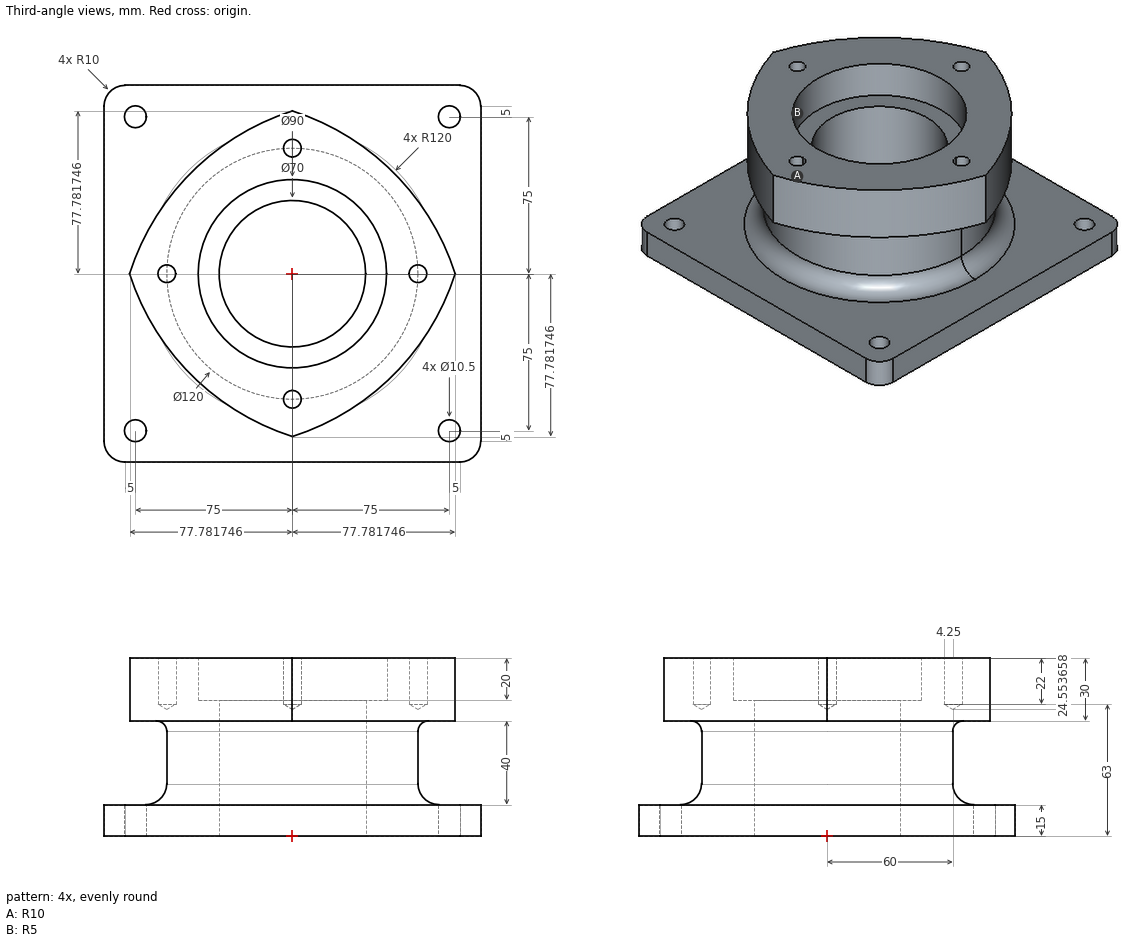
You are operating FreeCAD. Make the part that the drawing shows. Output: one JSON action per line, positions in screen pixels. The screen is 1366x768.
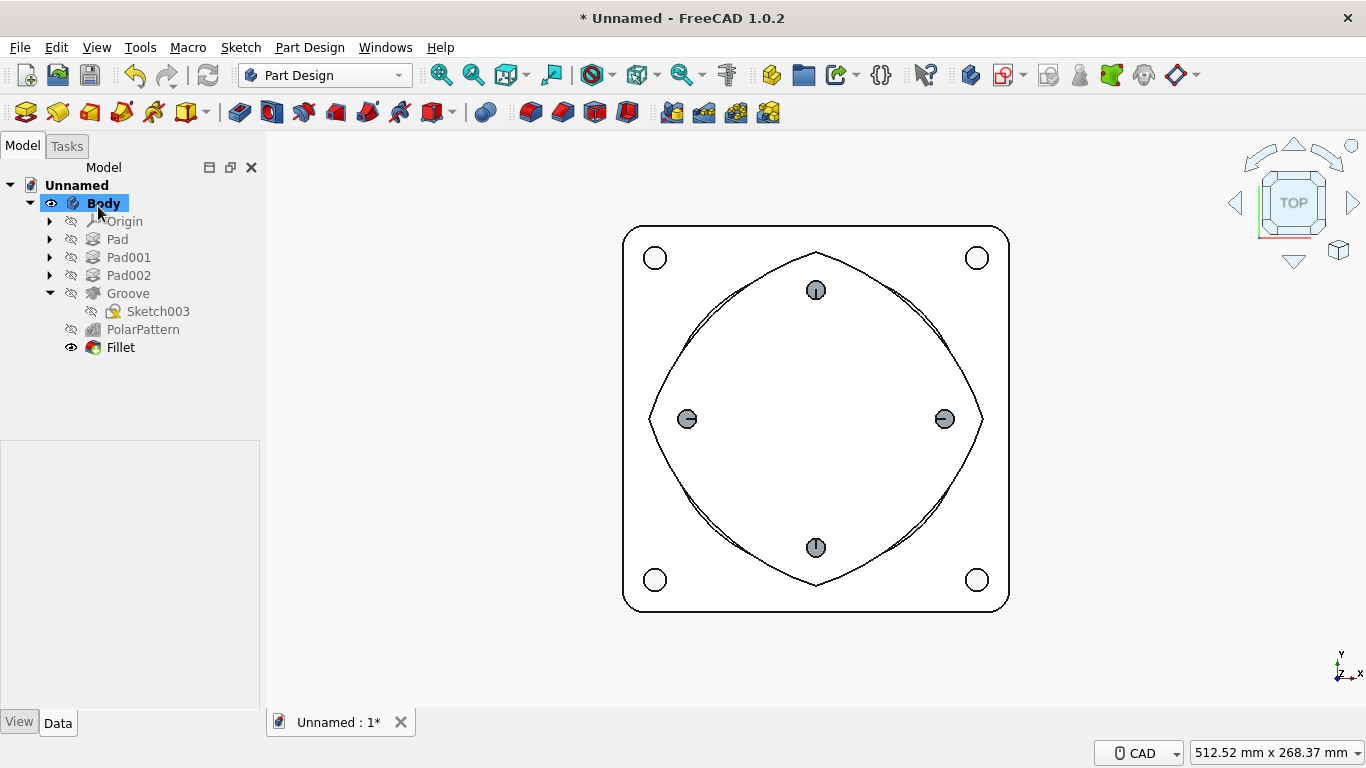
{"action": "key", "text": "0"}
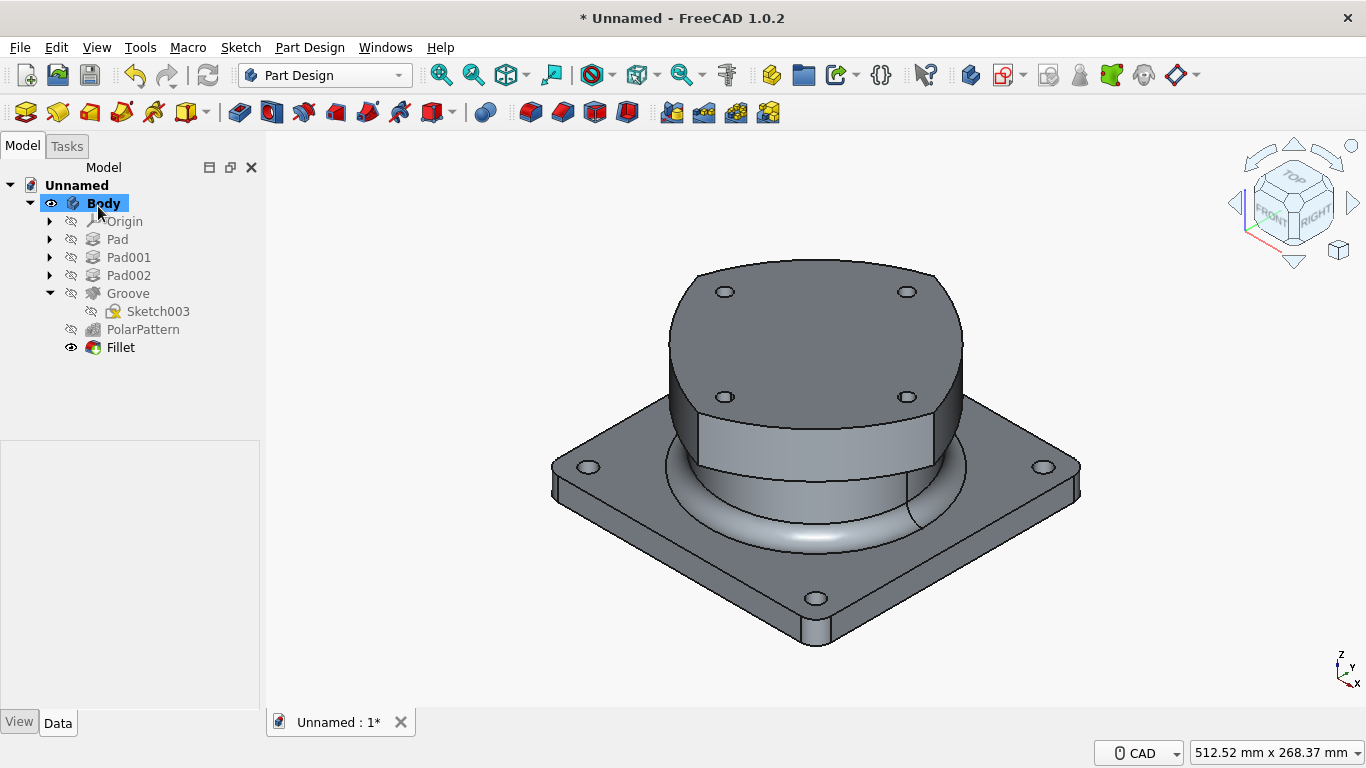
{"action": "key", "text": "1"}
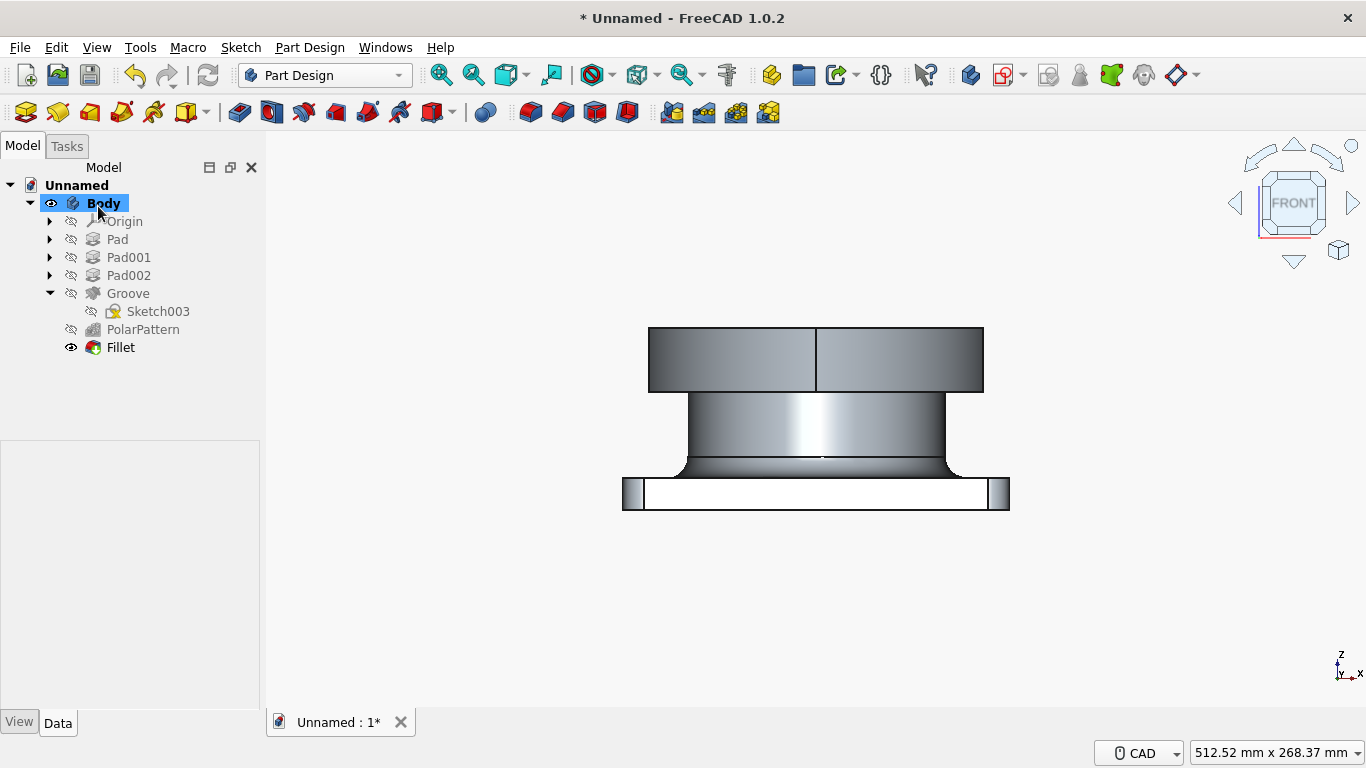
{"action": "left_click", "coordinate": [442, 76]}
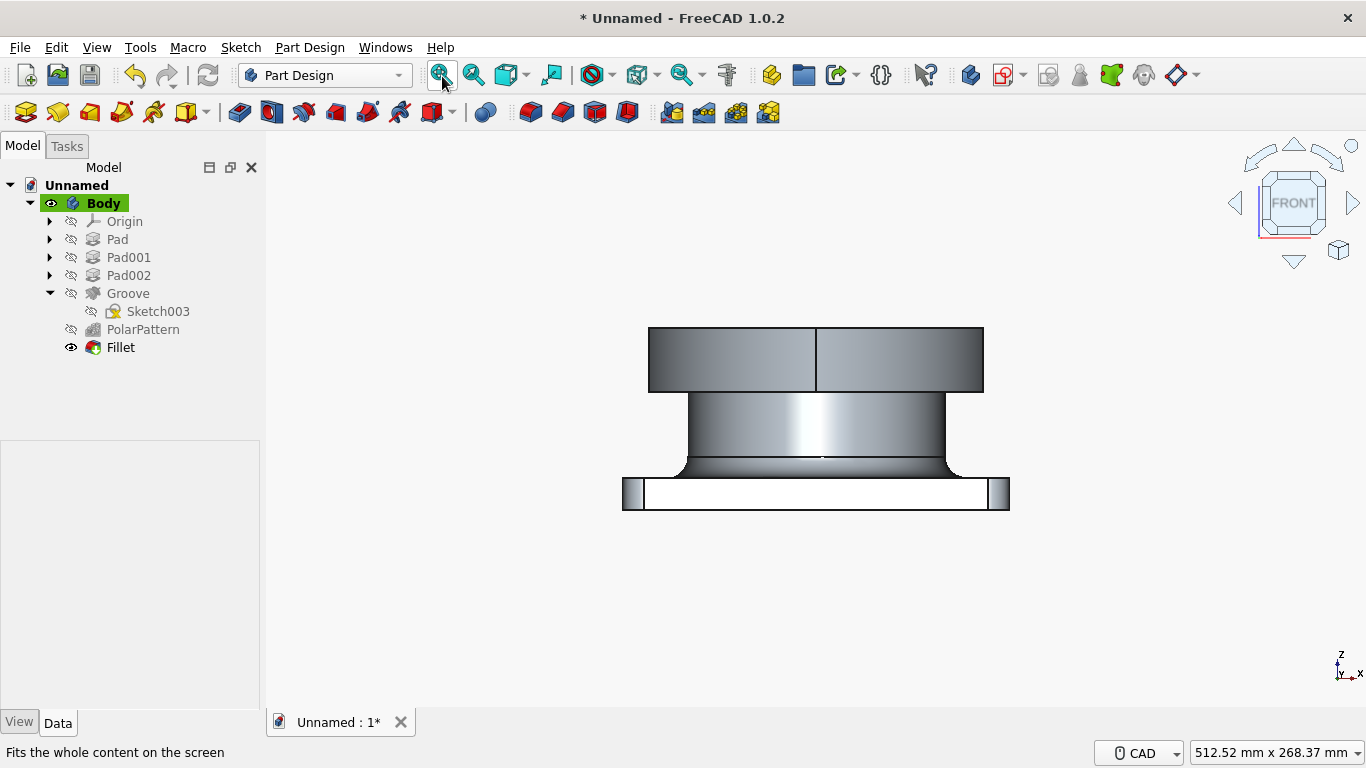
{"action": "key", "text": "3"}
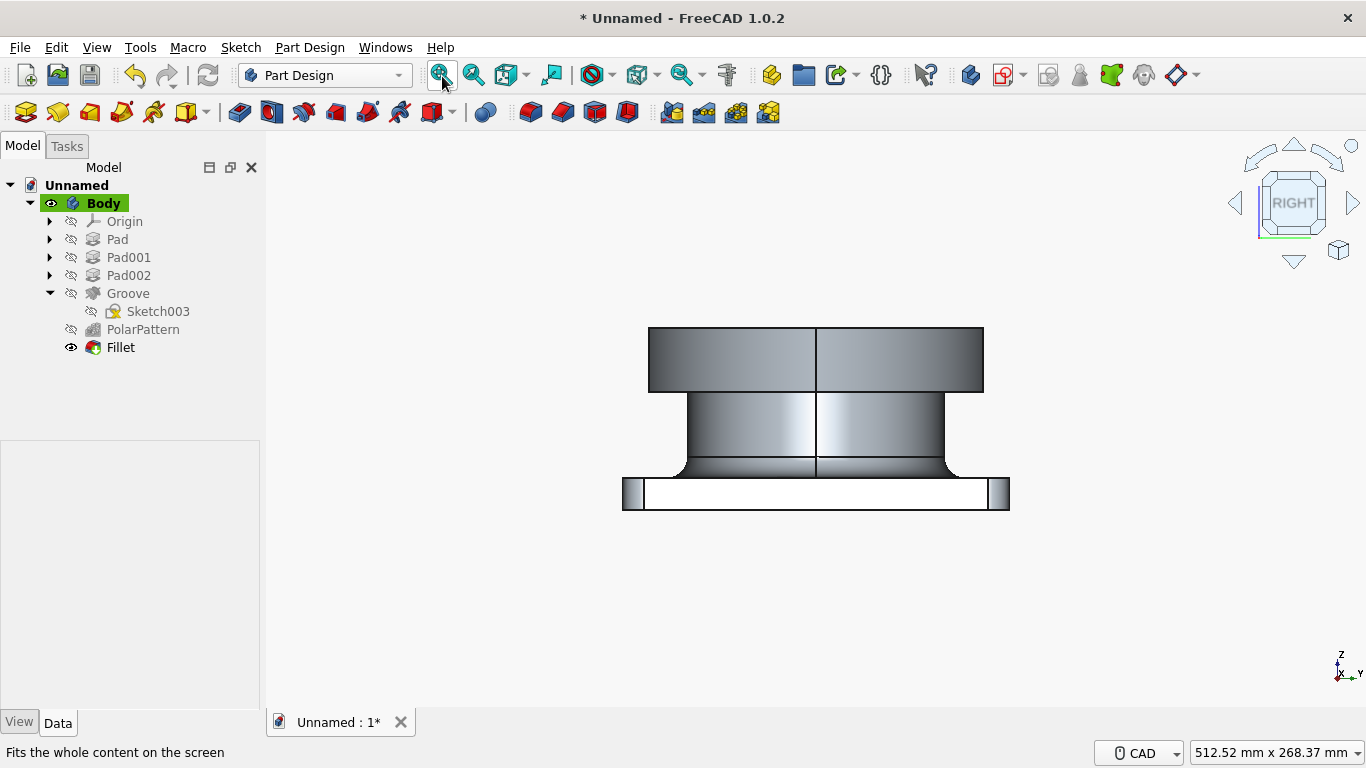
{"action": "left_click", "coordinate": [442, 76]}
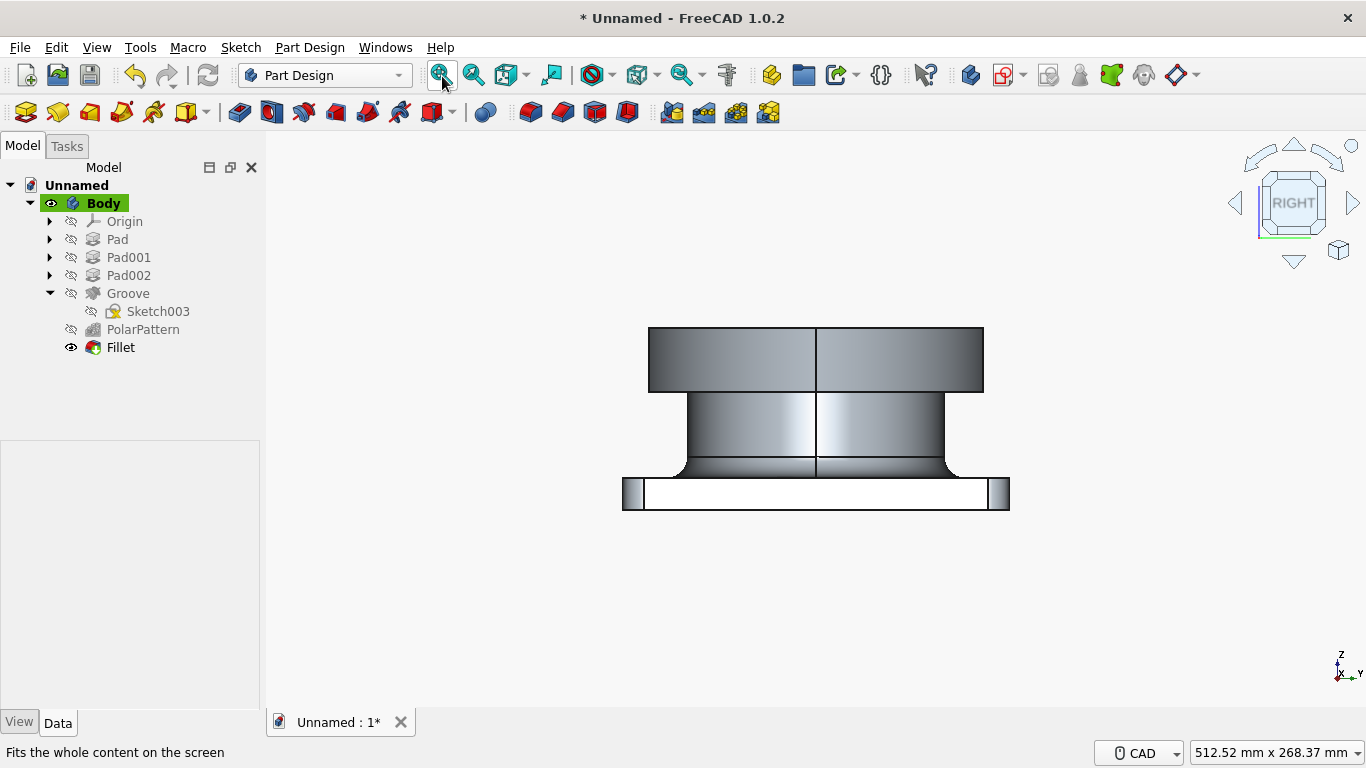
{"action": "key", "text": "5"}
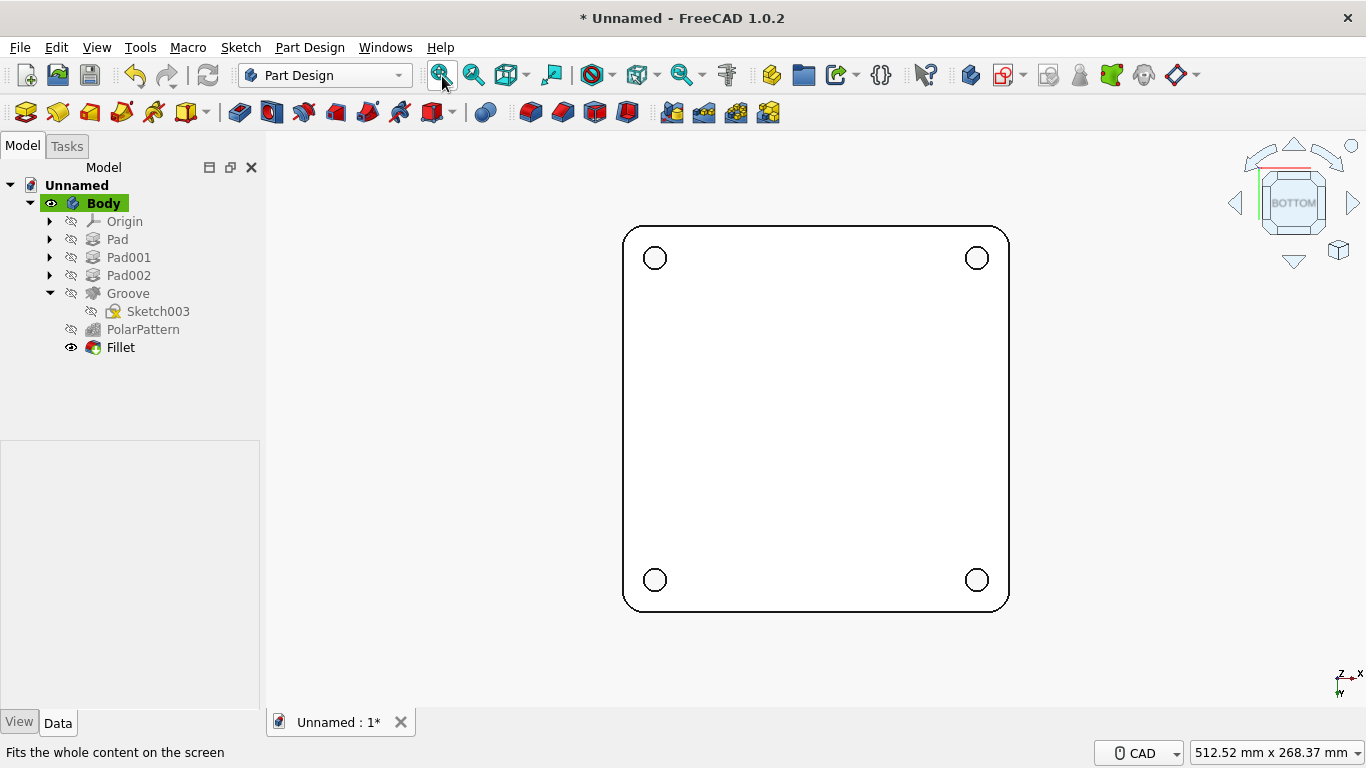
{"action": "key", "text": "4"}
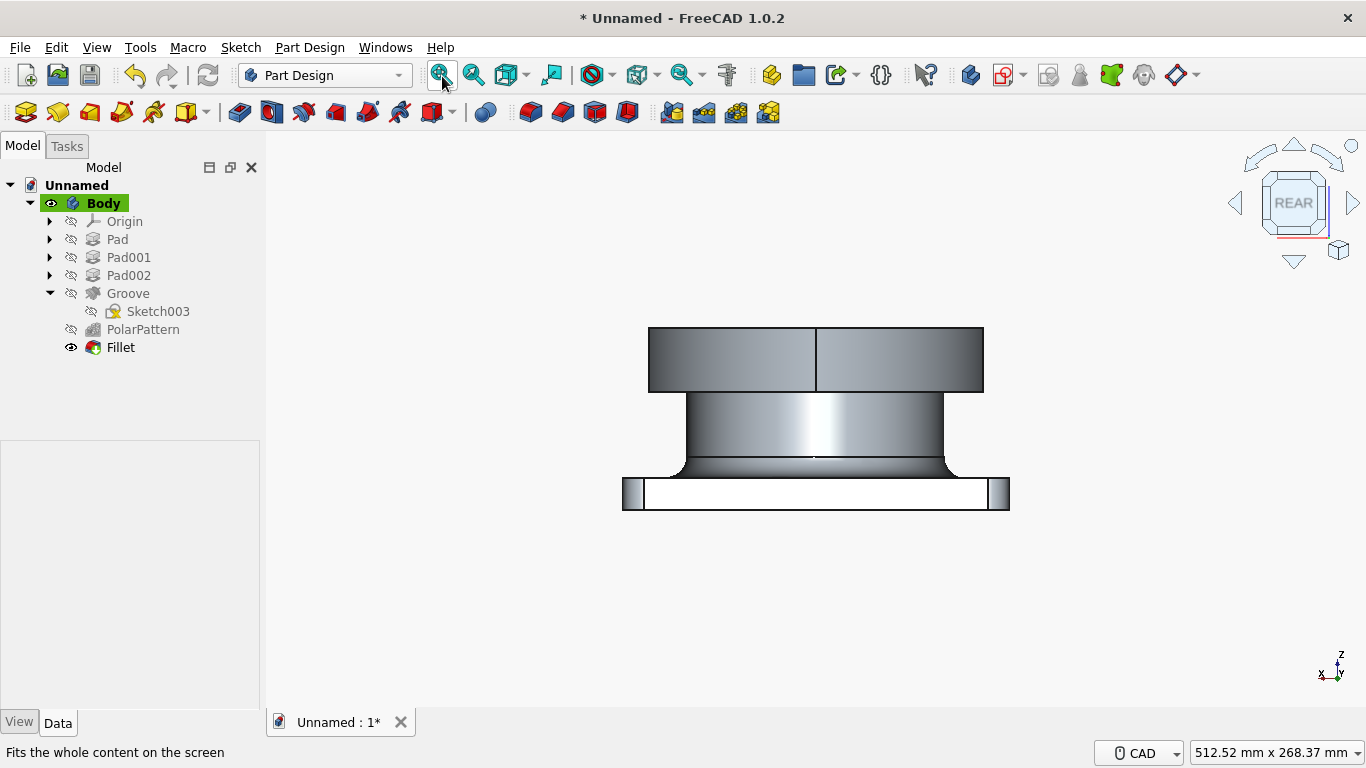
{"action": "left_click", "coordinate": [442, 76]}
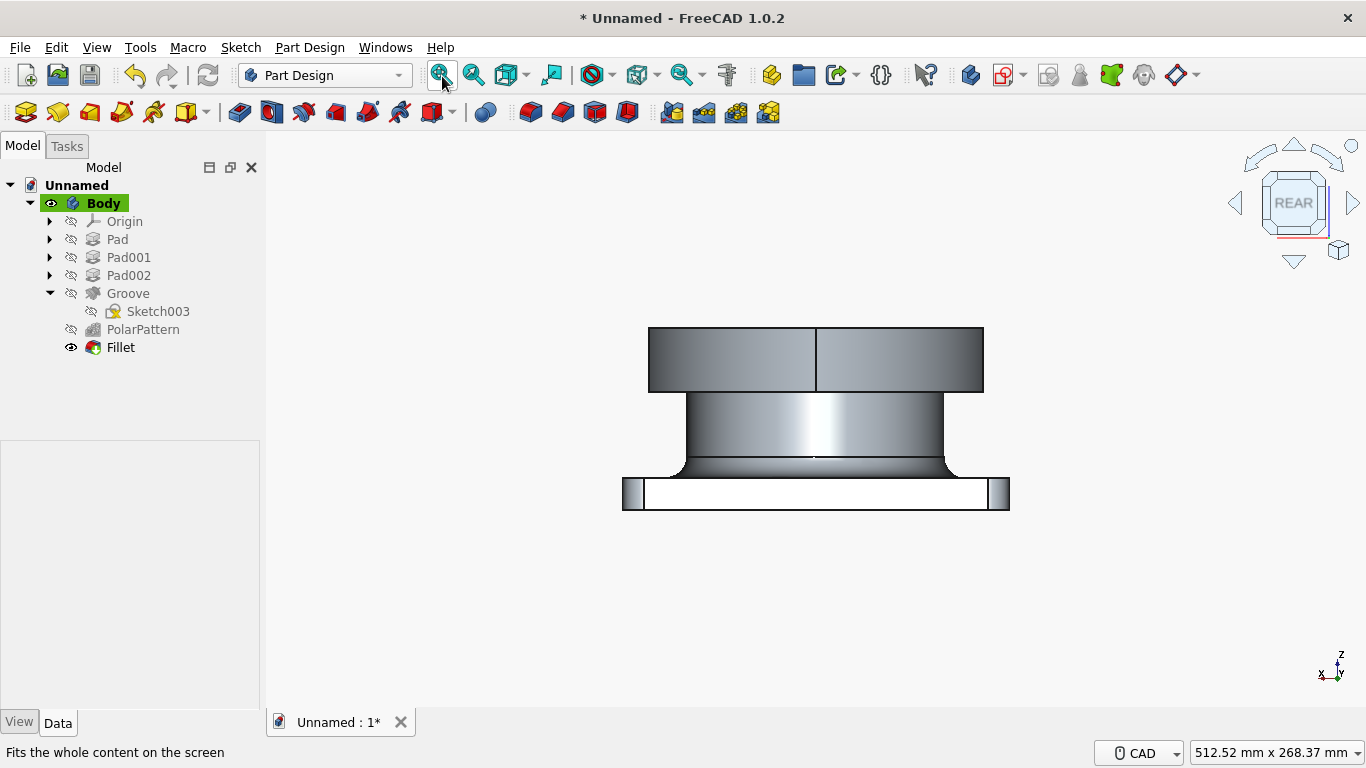
{"action": "key", "text": "6"}